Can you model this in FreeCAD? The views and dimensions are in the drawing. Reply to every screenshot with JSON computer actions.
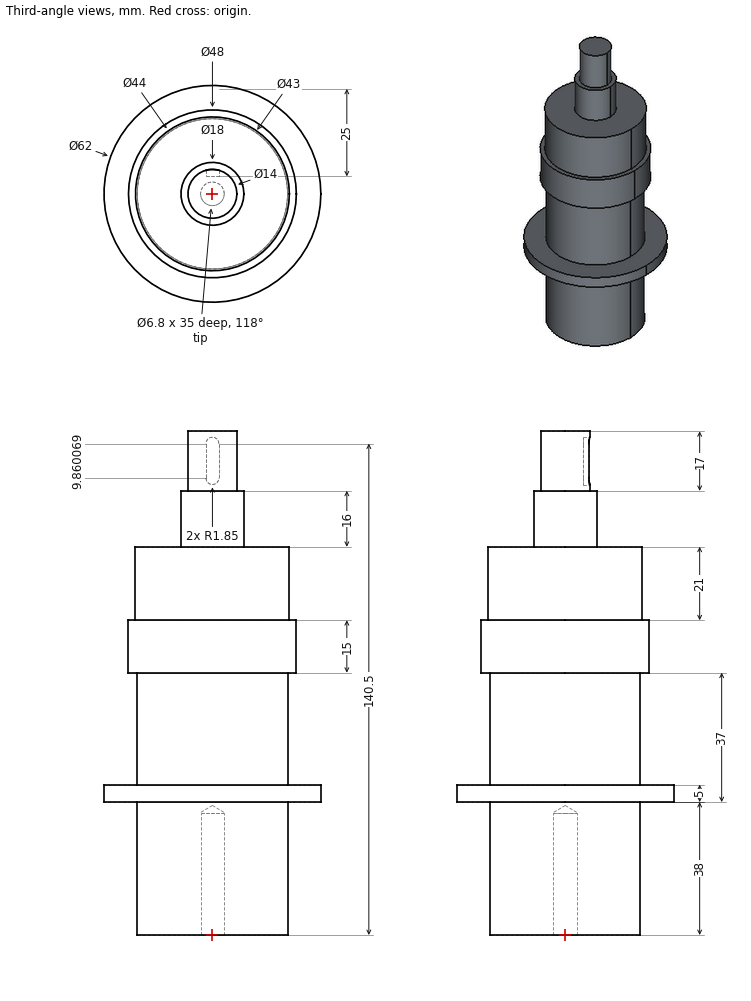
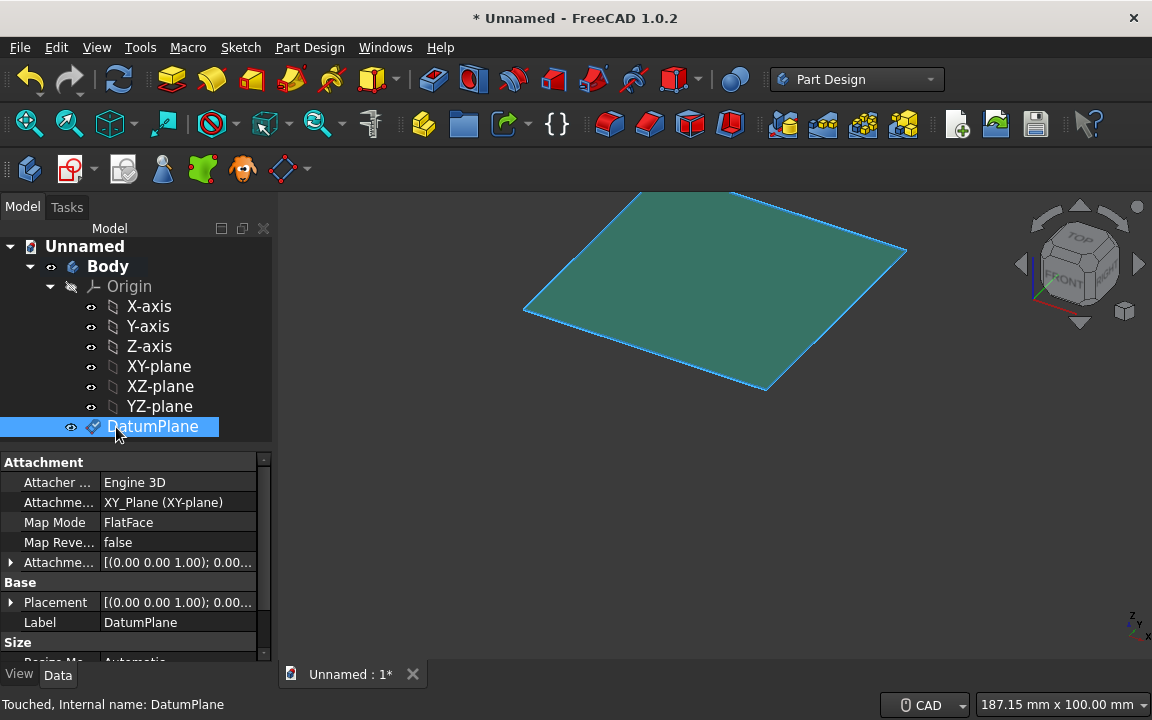
{"action": "left_click", "coordinate": [70, 170]}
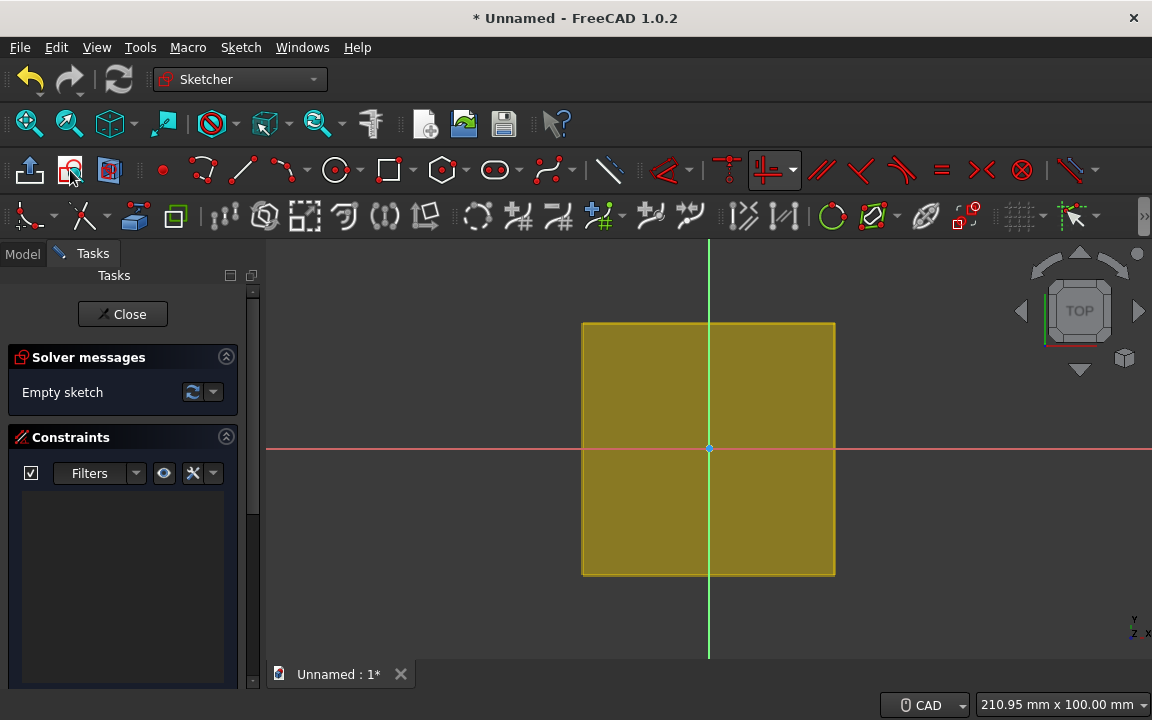
{"action": "scroll", "coordinate": [848, 449], "scroll_direction": "up", "scroll_amount": 2}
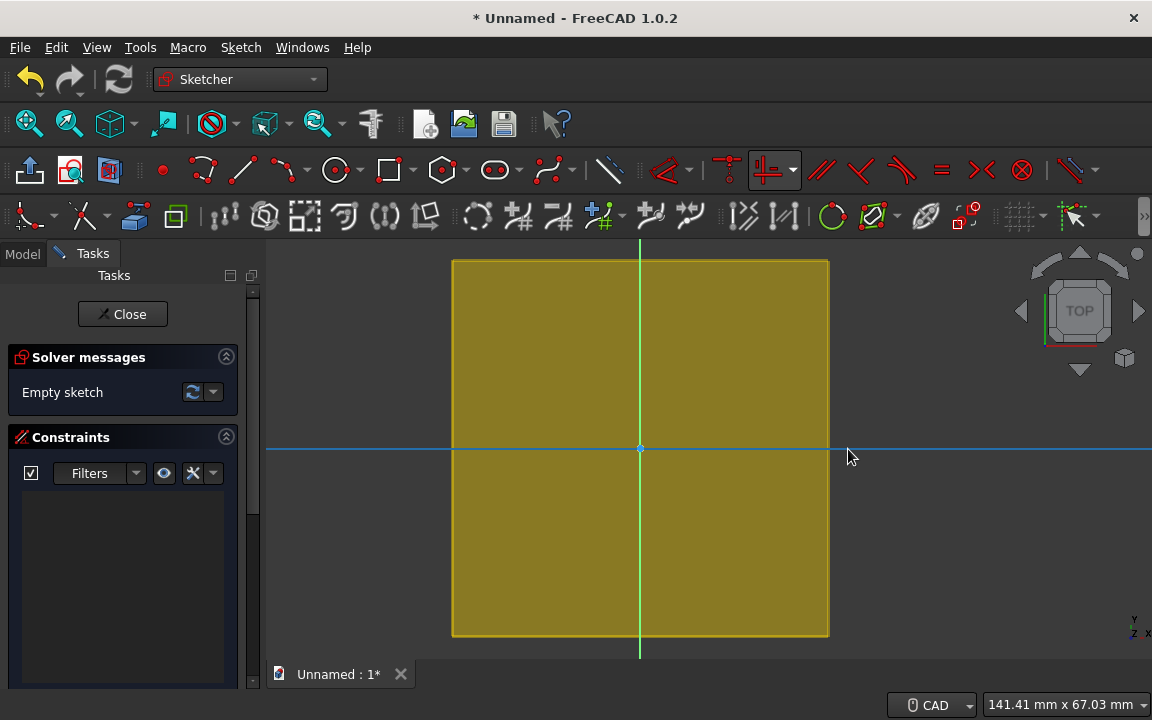
{"action": "key", "text": "g c"}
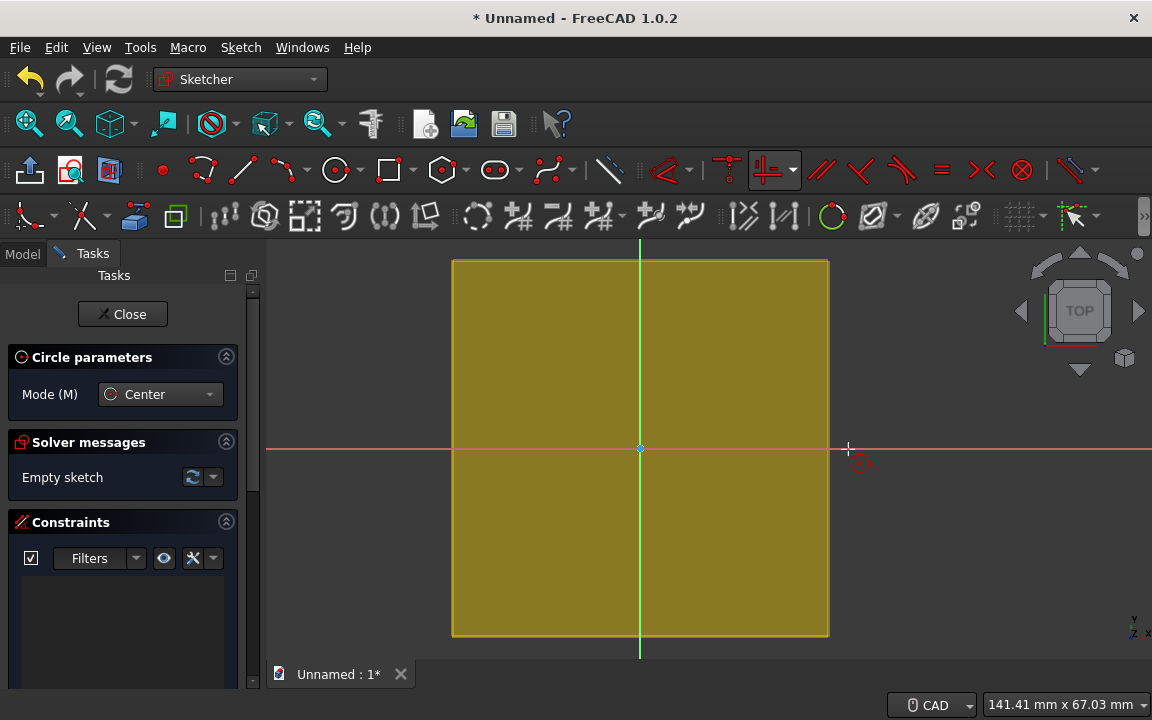
{"action": "left_click", "coordinate": [640, 449]}
{"action": "left_click", "coordinate": [736, 353]}
{"action": "key", "text": "Escape"}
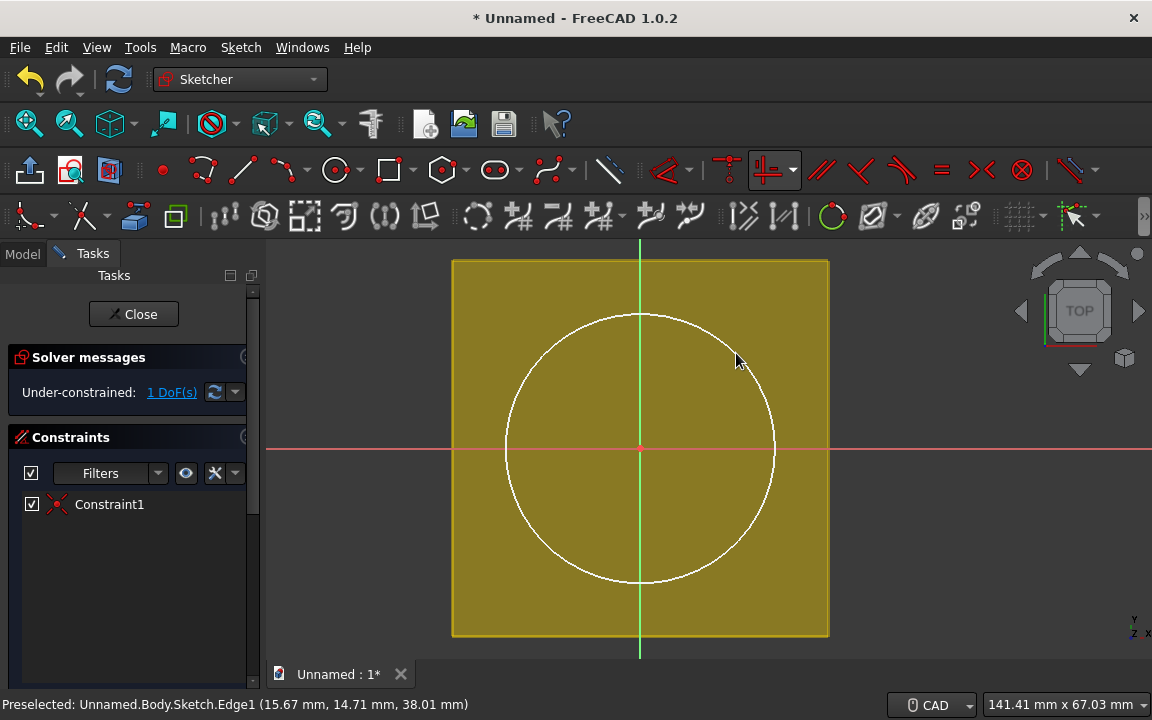
{"action": "left_click", "coordinate": [664, 170]}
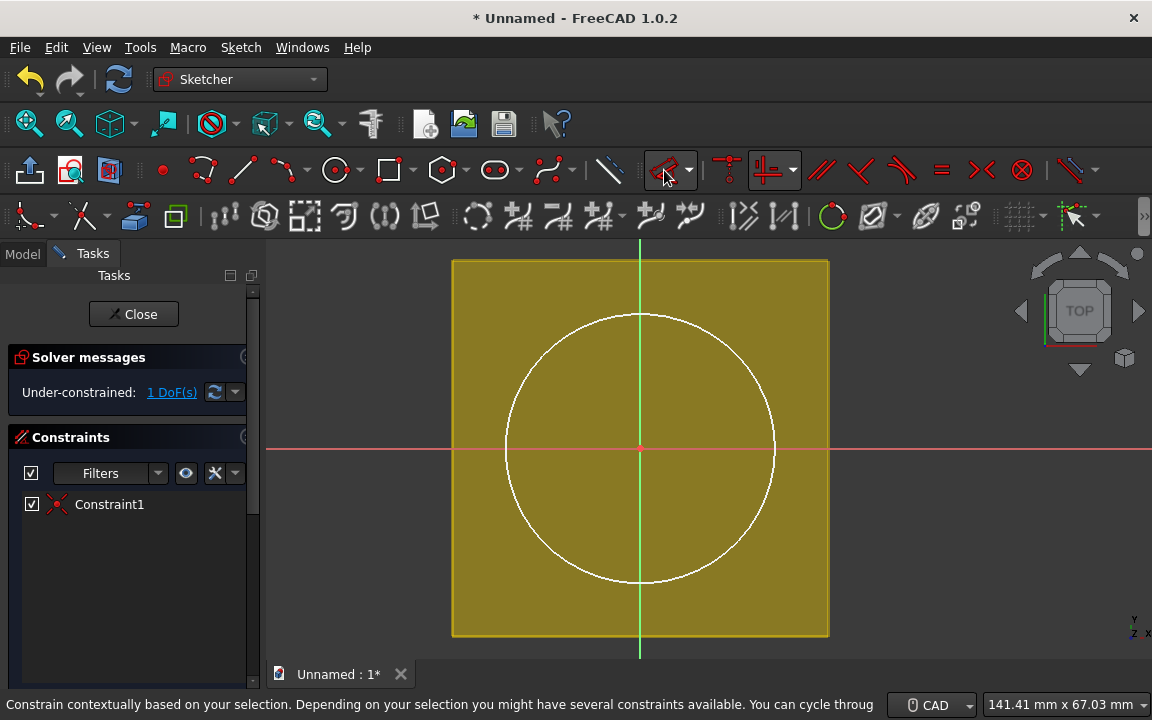
{"action": "left_click", "coordinate": [735, 353]}
{"action": "left_click", "coordinate": [758, 330]}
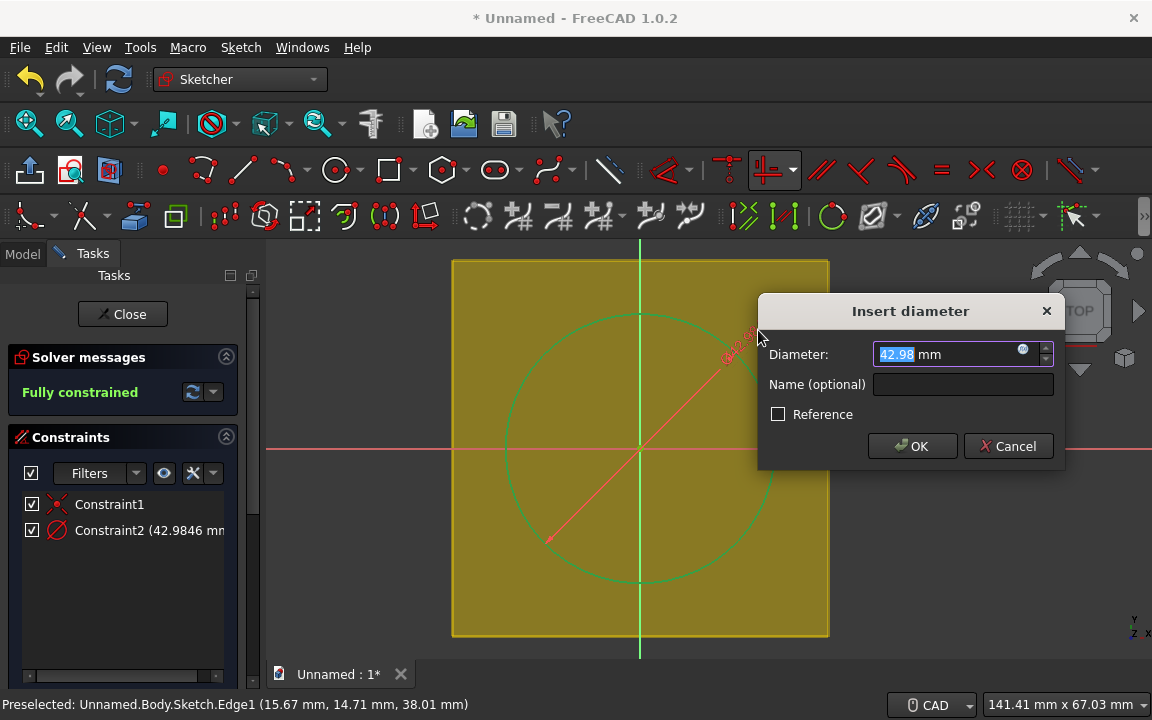
{"action": "type", "text": "43"}
{"action": "key", "text": "Return"}
{"action": "key", "text": "Escape"}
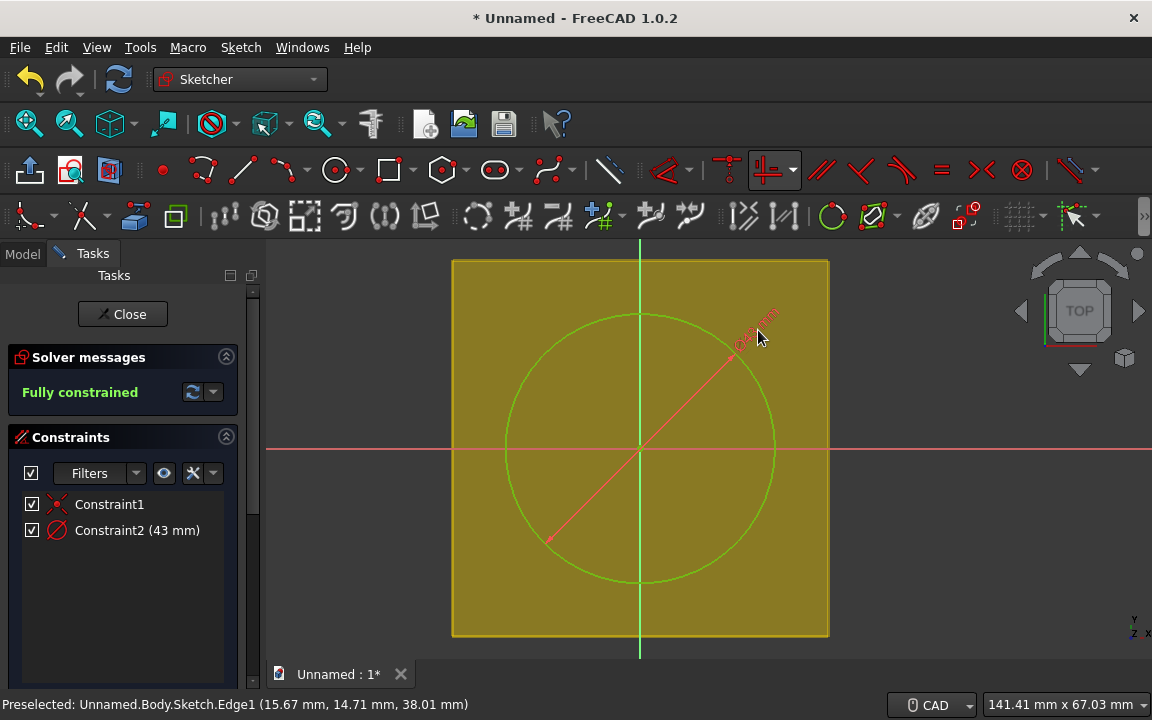
{"action": "left_click", "coordinate": [123, 314]}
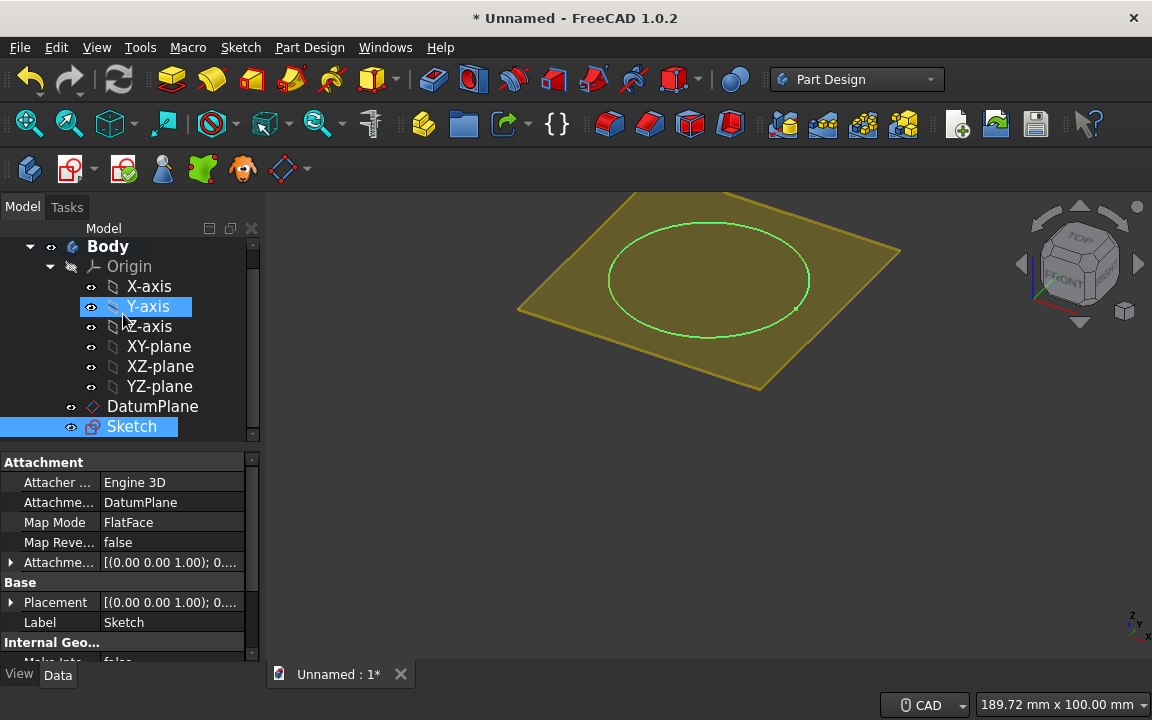
{"action": "left_click", "coordinate": [172, 80]}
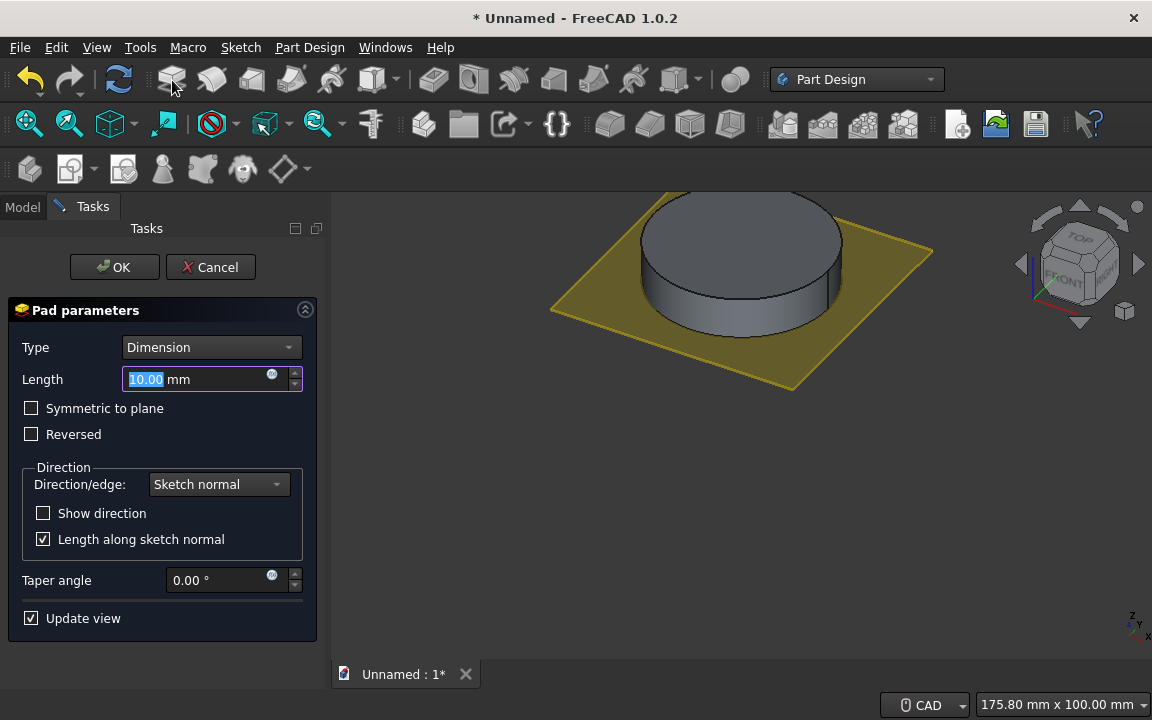
{"action": "type", "text": "37"}
{"action": "key", "text": "Tab"}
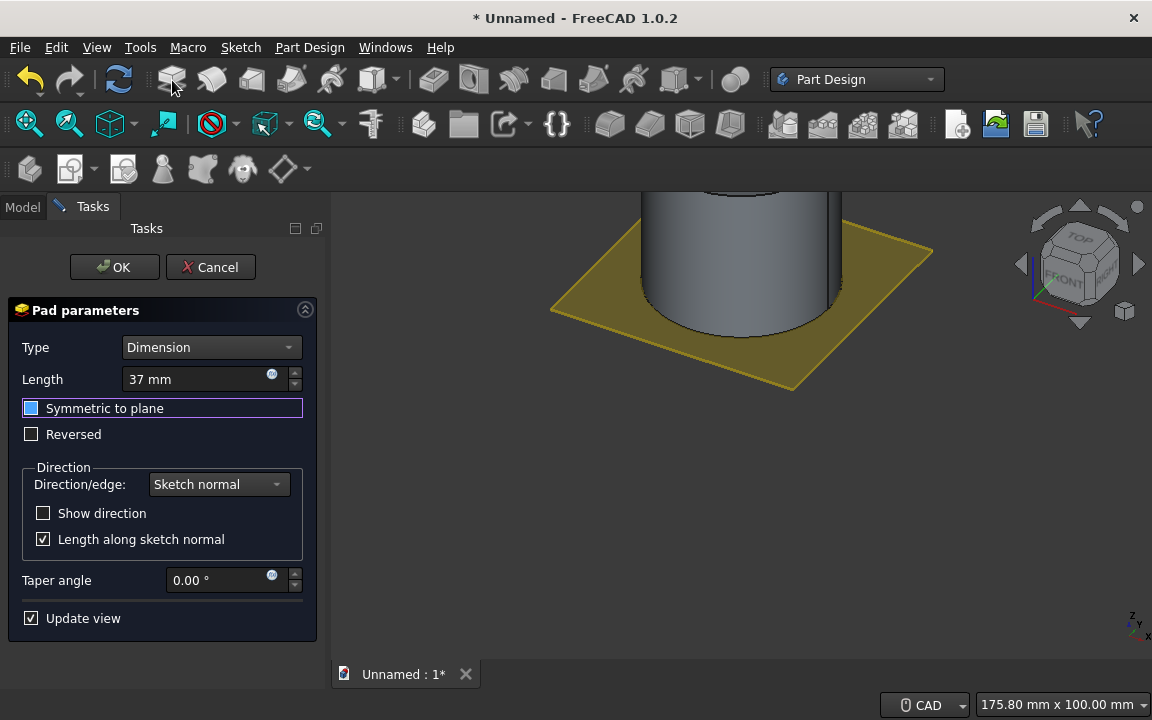
{"action": "left_click", "coordinate": [115, 267]}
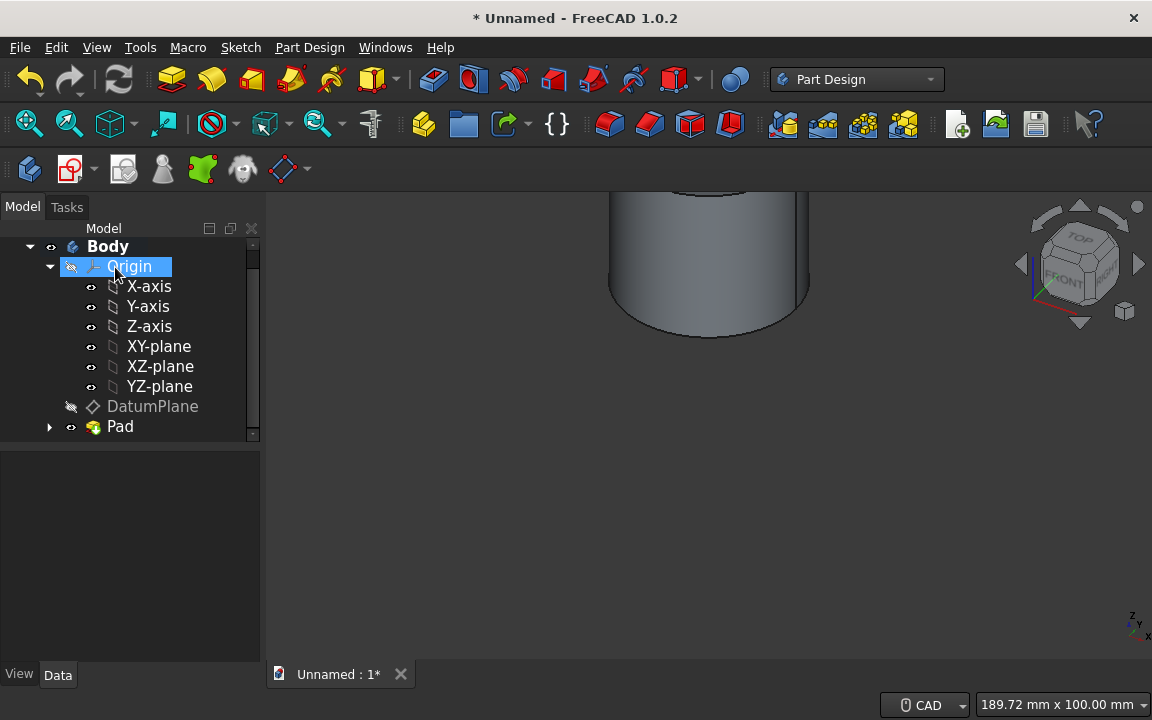
{"action": "left_click", "coordinate": [30, 124]}